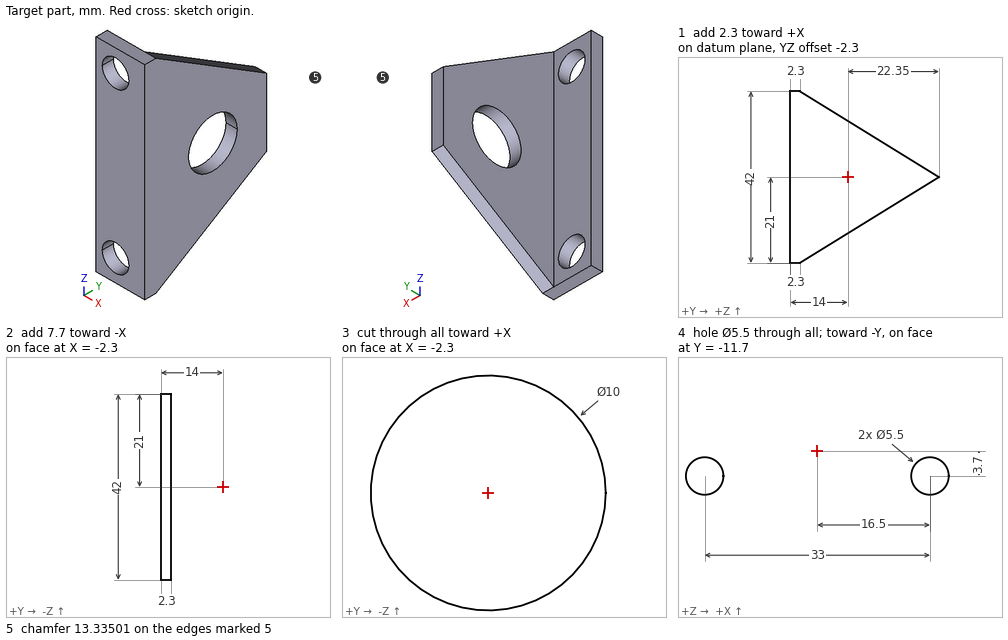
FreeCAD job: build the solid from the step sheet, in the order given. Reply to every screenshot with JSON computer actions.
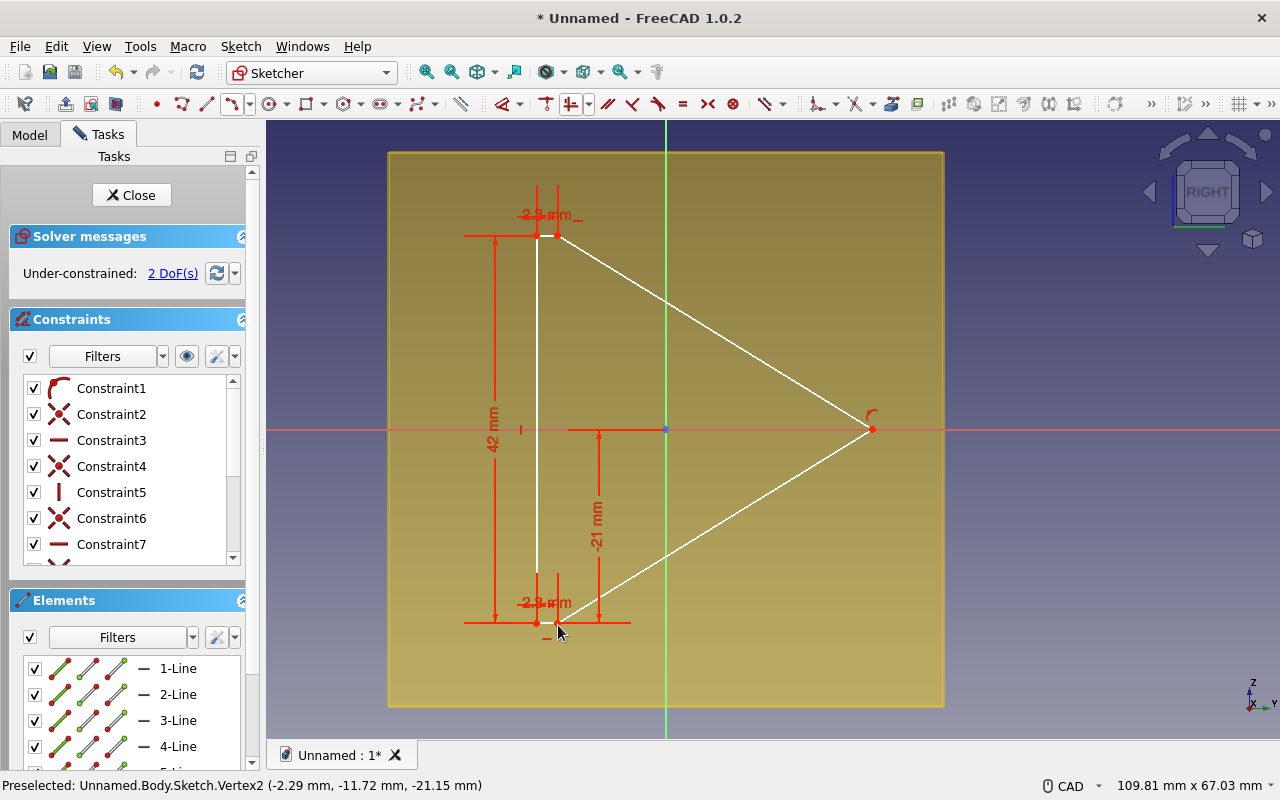
{"action": "left_click", "coordinate": [537, 623]}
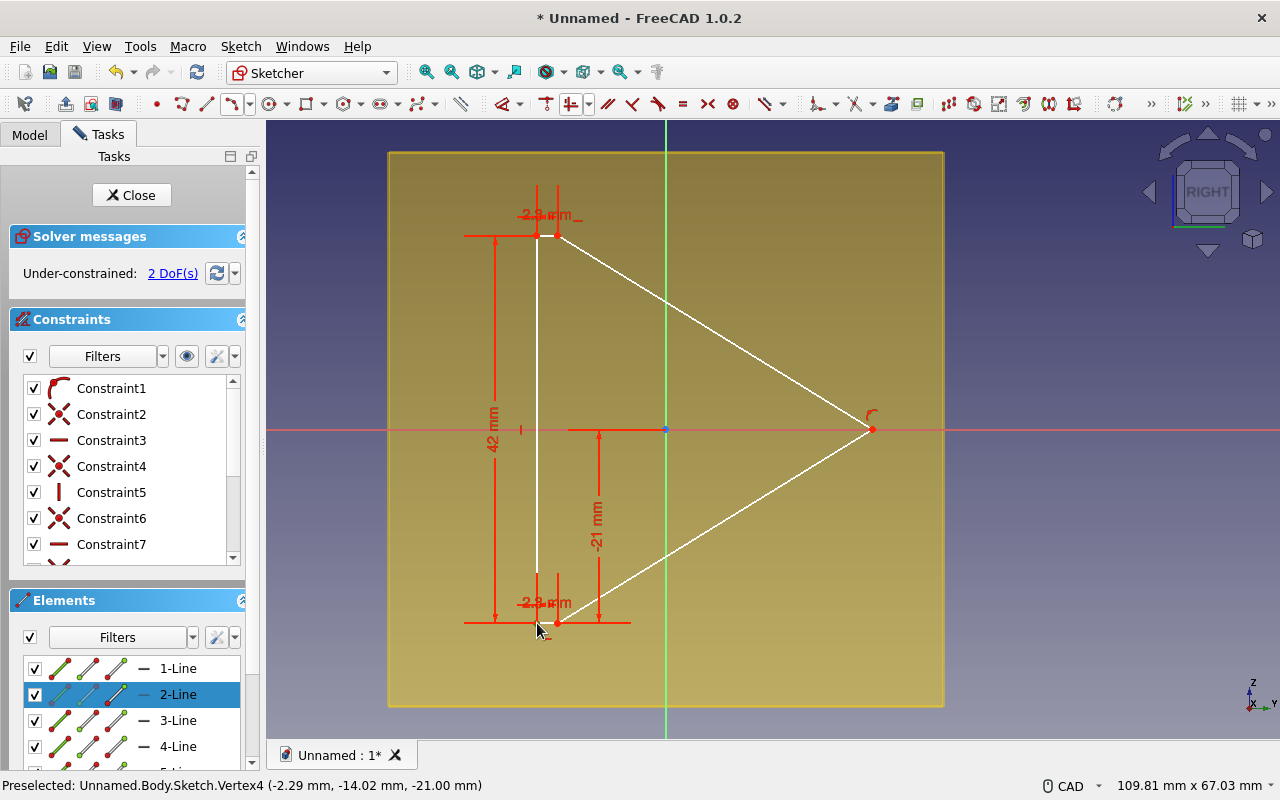
{"action": "left_click", "coordinate": [520, 104]}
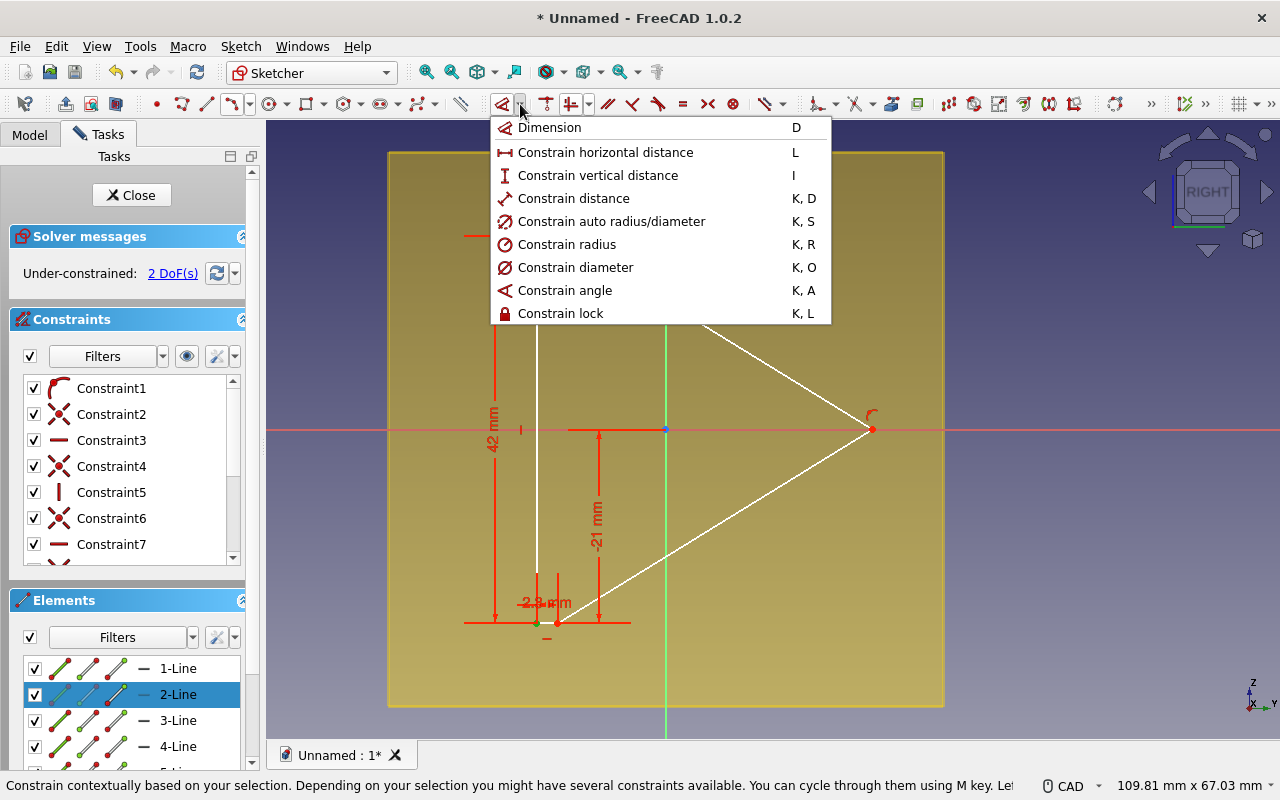
{"action": "left_click", "coordinate": [661, 152]}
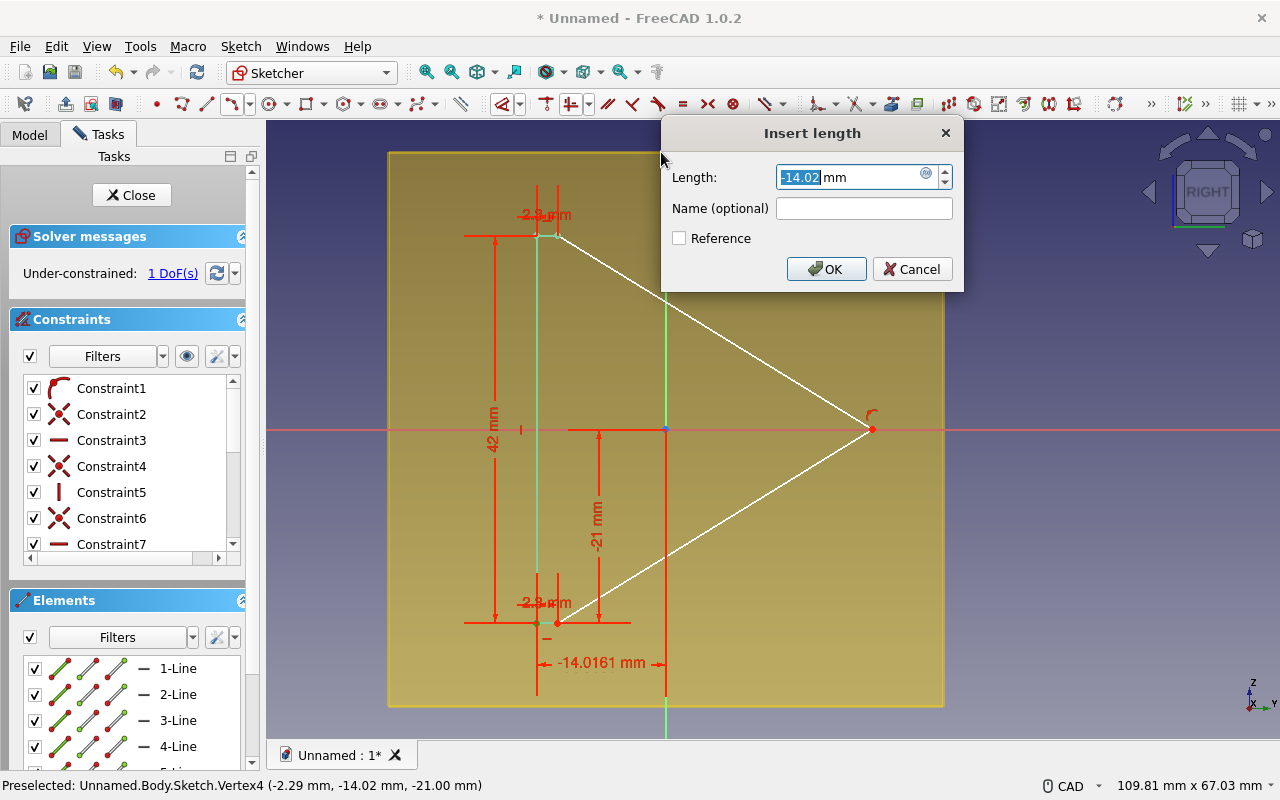
{"action": "type", "text": "-14"}
{"action": "key", "text": "Return"}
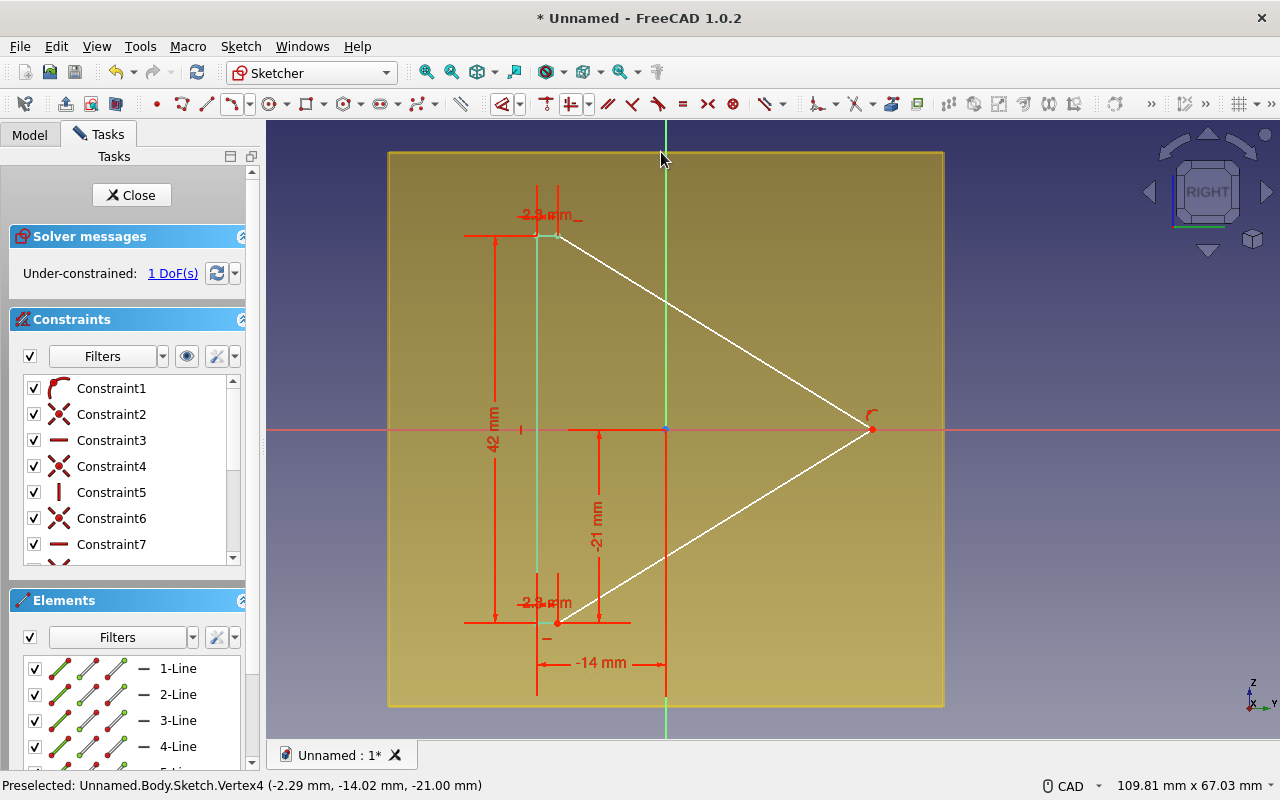
{"action": "left_click", "coordinate": [873, 429]}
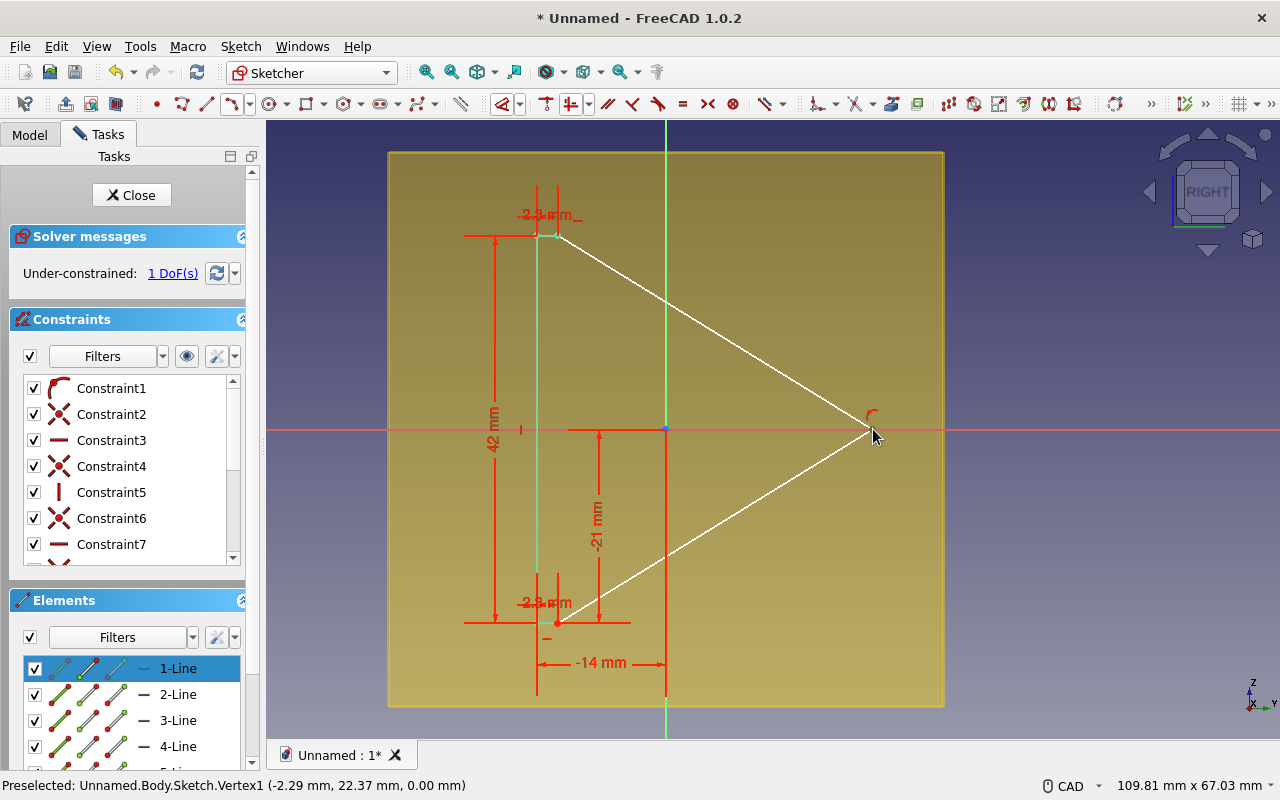
{"action": "key", "text": "l"}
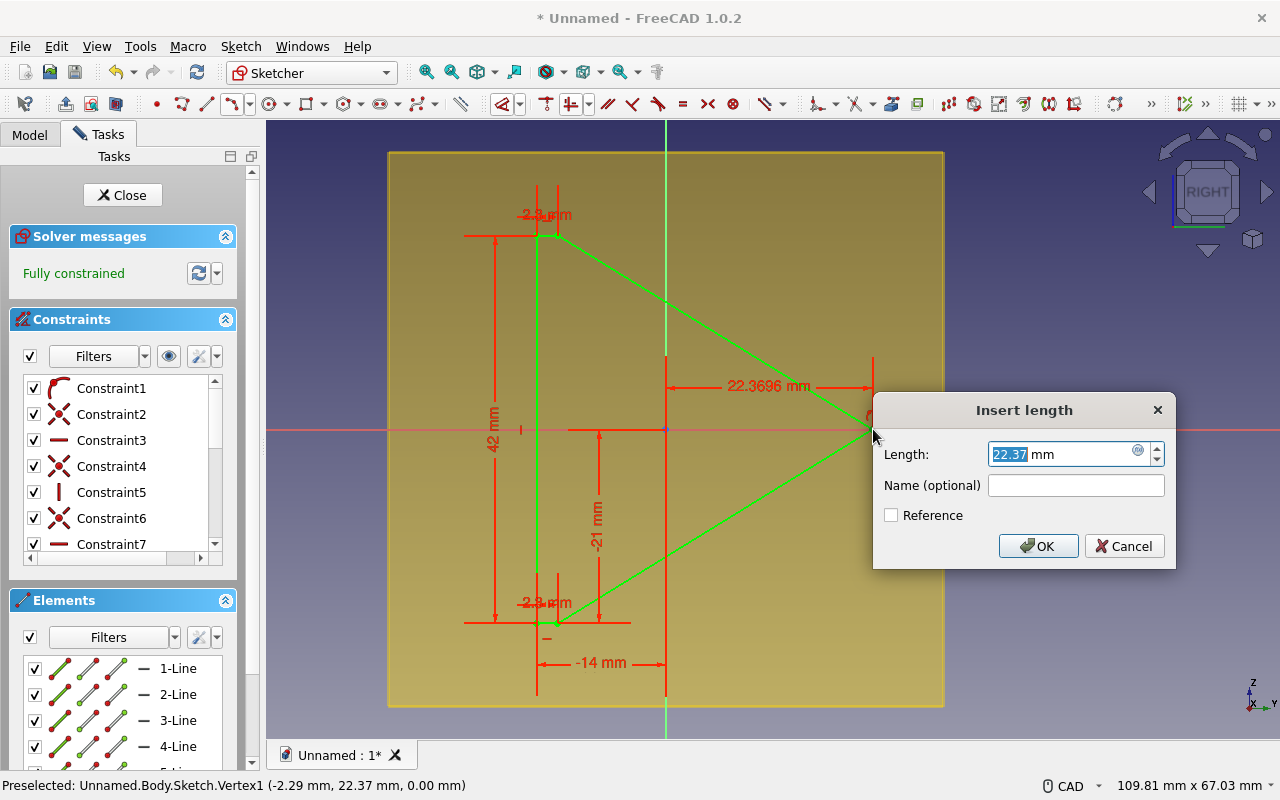
{"action": "type", "text": "22.35"}
{"action": "key", "text": "Return"}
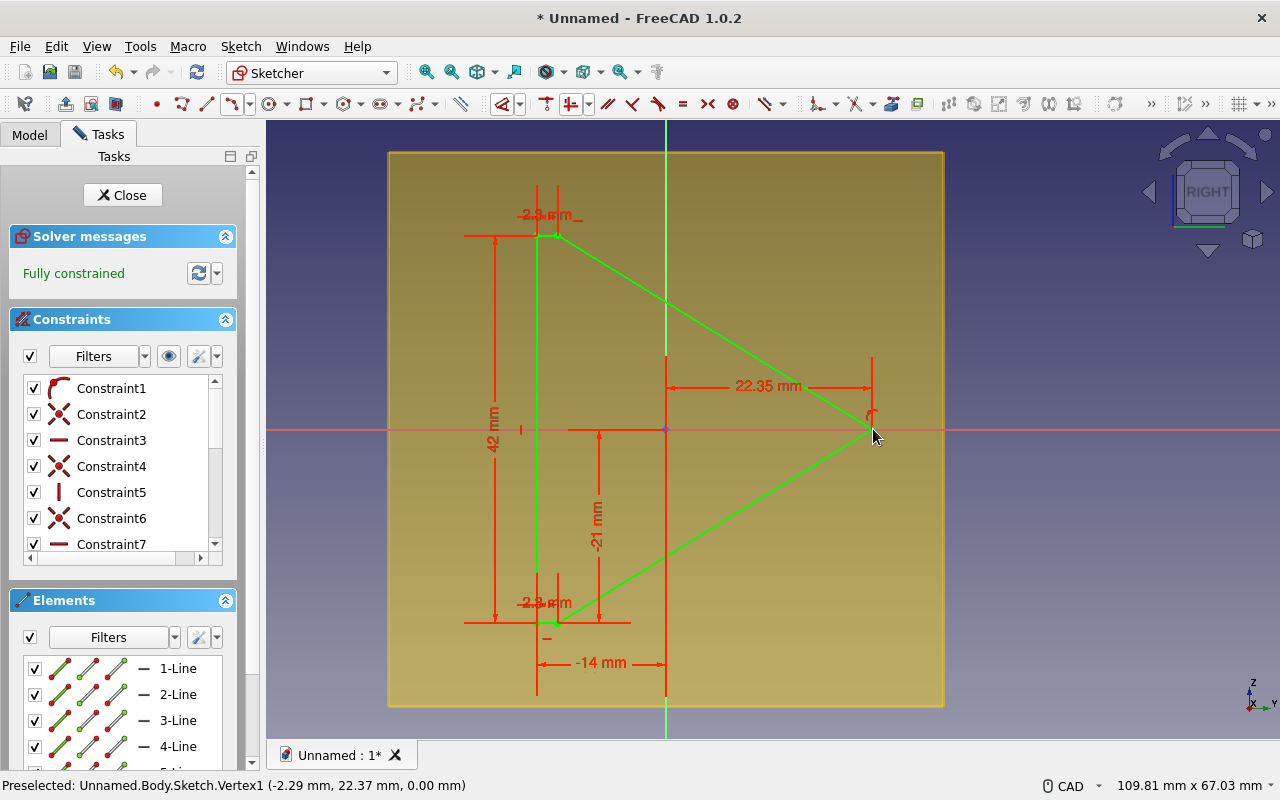
{"action": "left_click", "coordinate": [123, 195]}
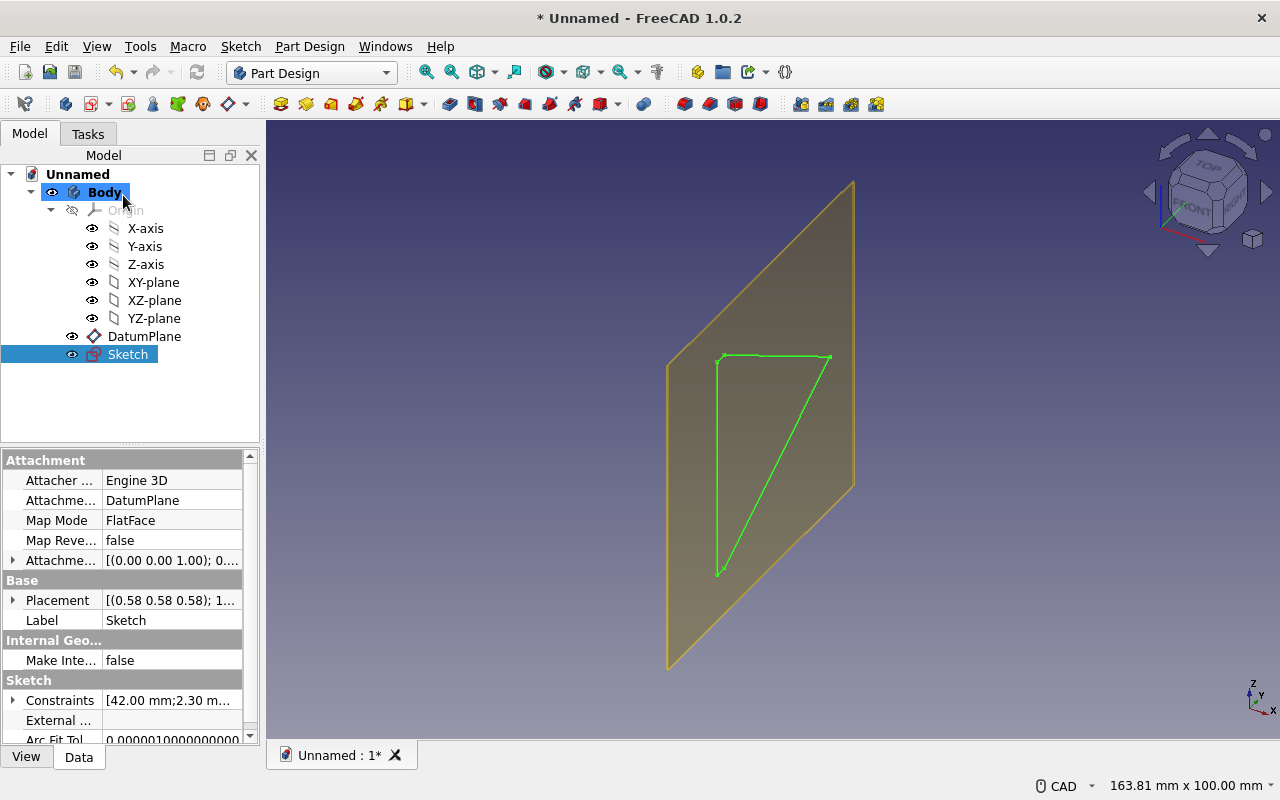
{"action": "left_click", "coordinate": [281, 104]}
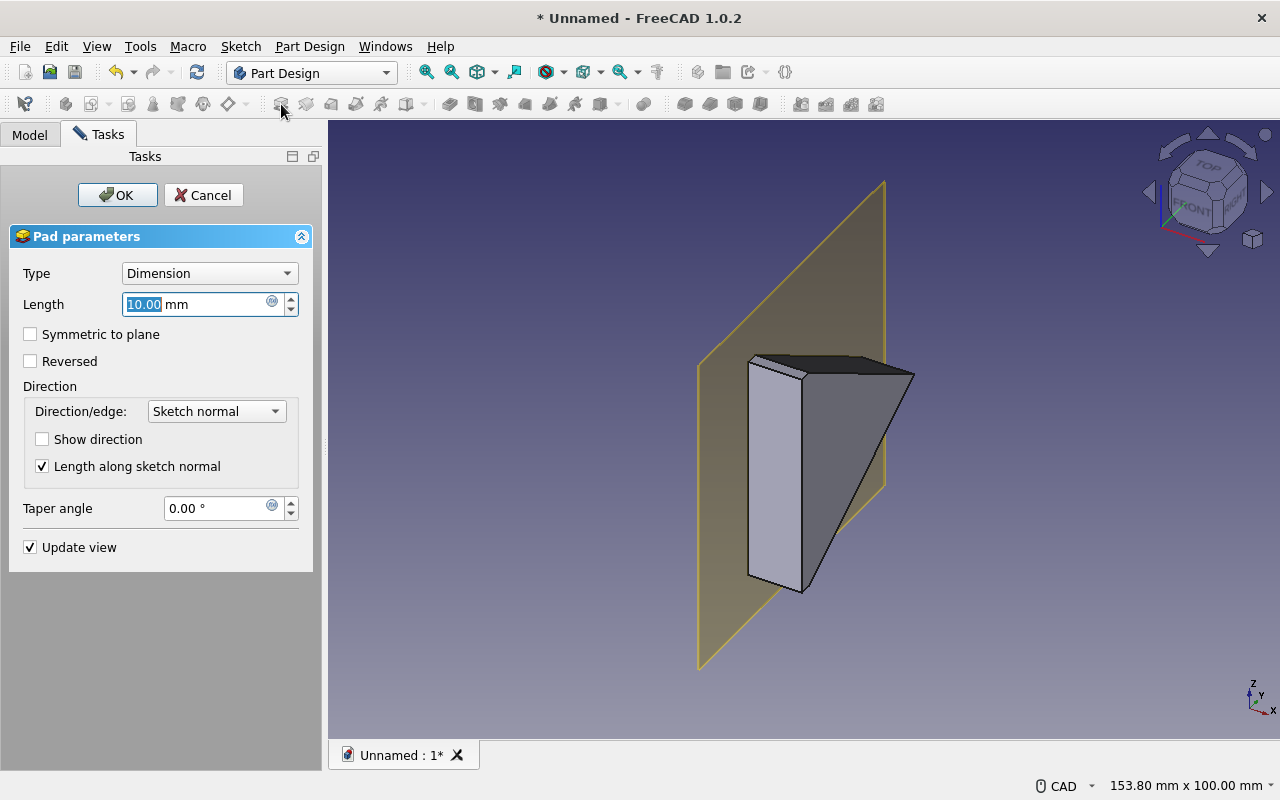
{"action": "type", "text": "2.3"}
{"action": "key", "text": "Tab"}